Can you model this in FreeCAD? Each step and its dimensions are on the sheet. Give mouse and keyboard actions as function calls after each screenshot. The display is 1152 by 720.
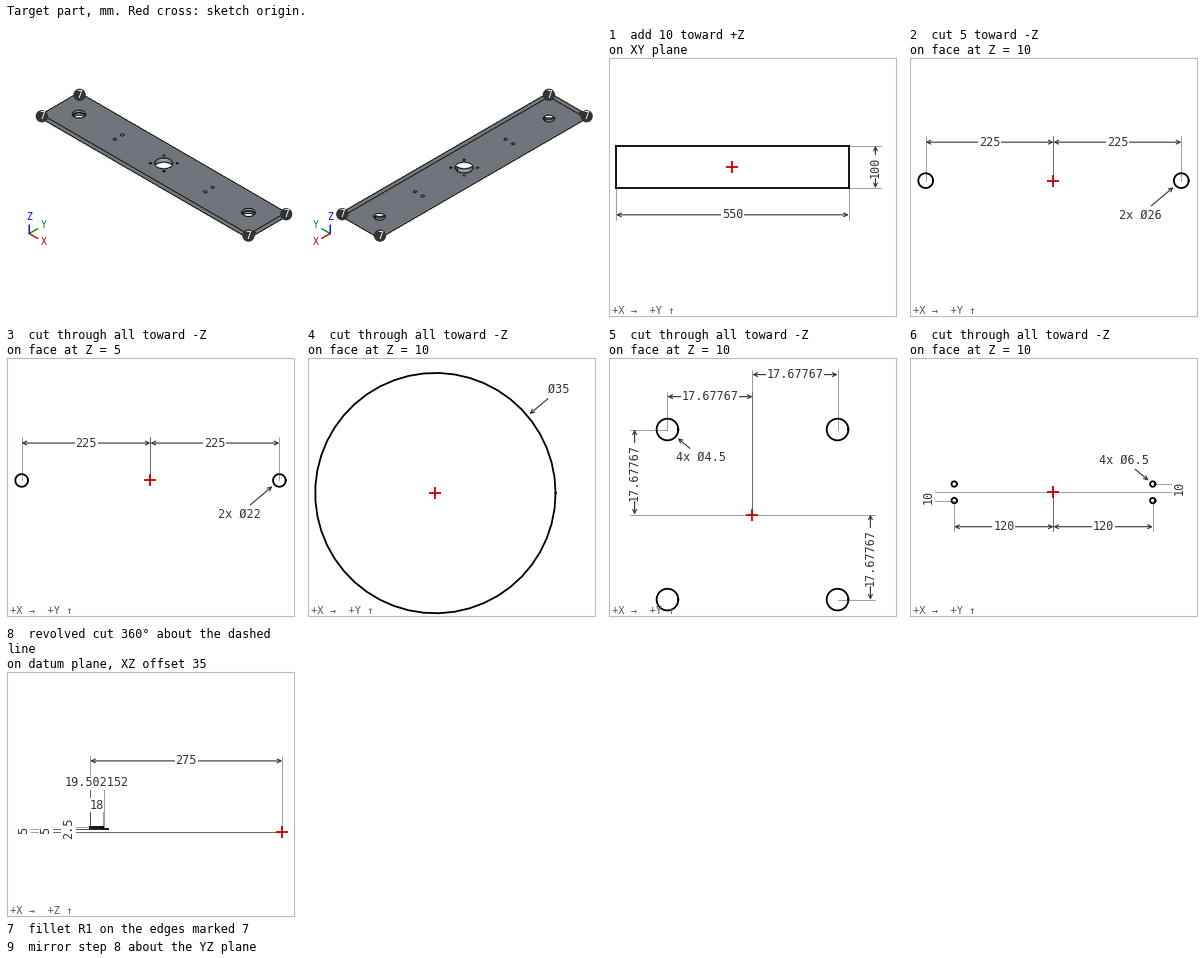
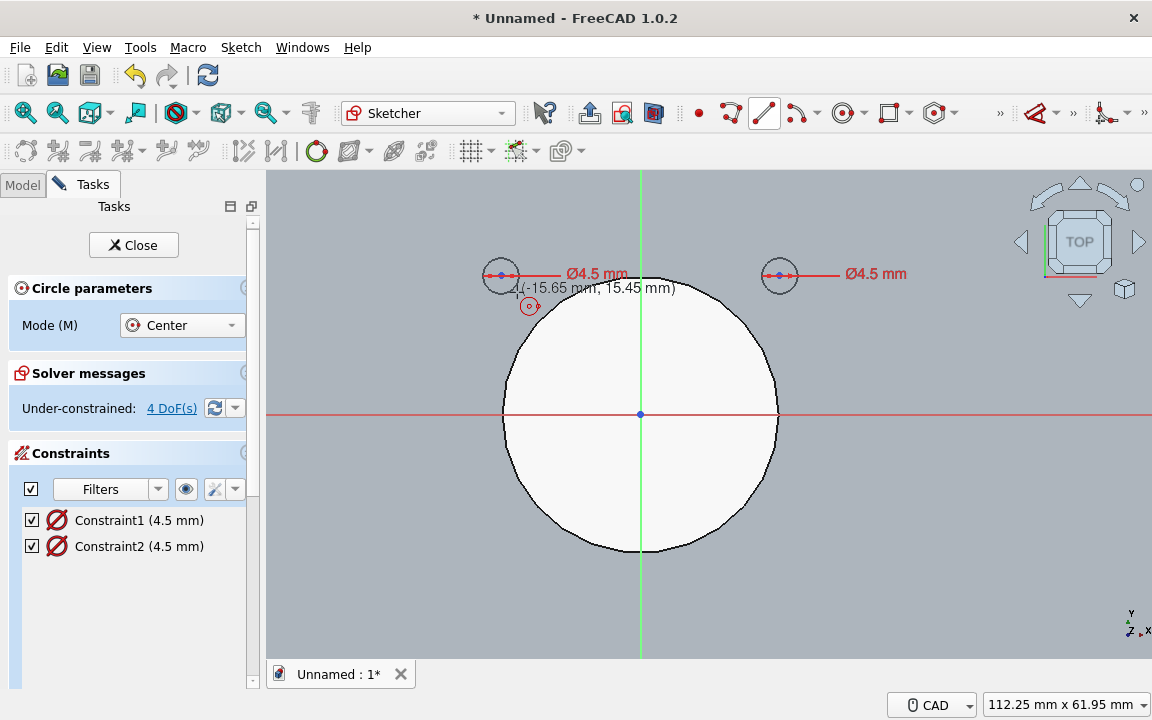
scroll(780, 554, up, 2)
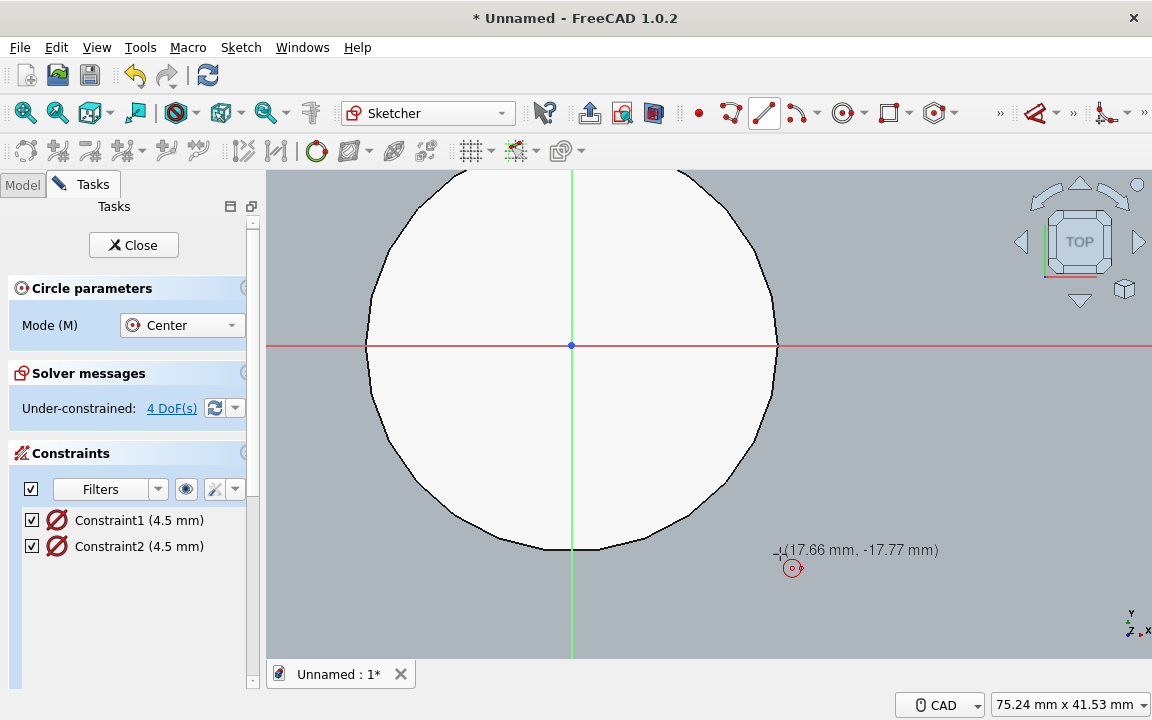
click(780, 554)
move(799, 535)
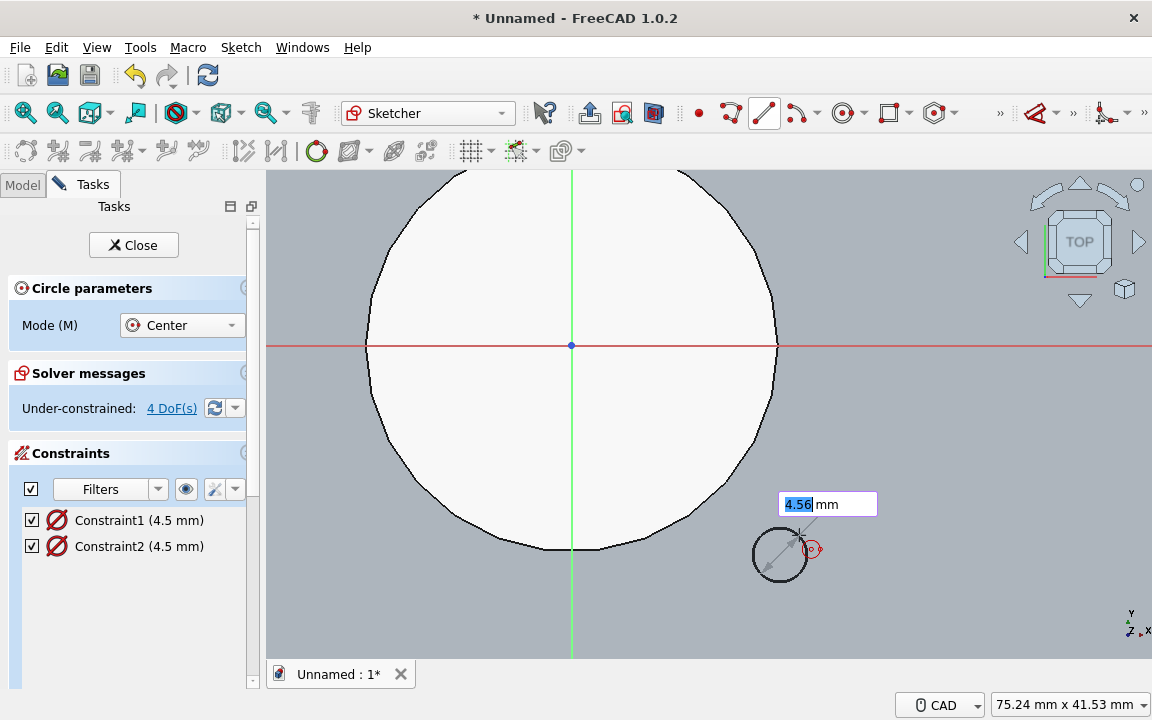
text(4.5)
key(Return)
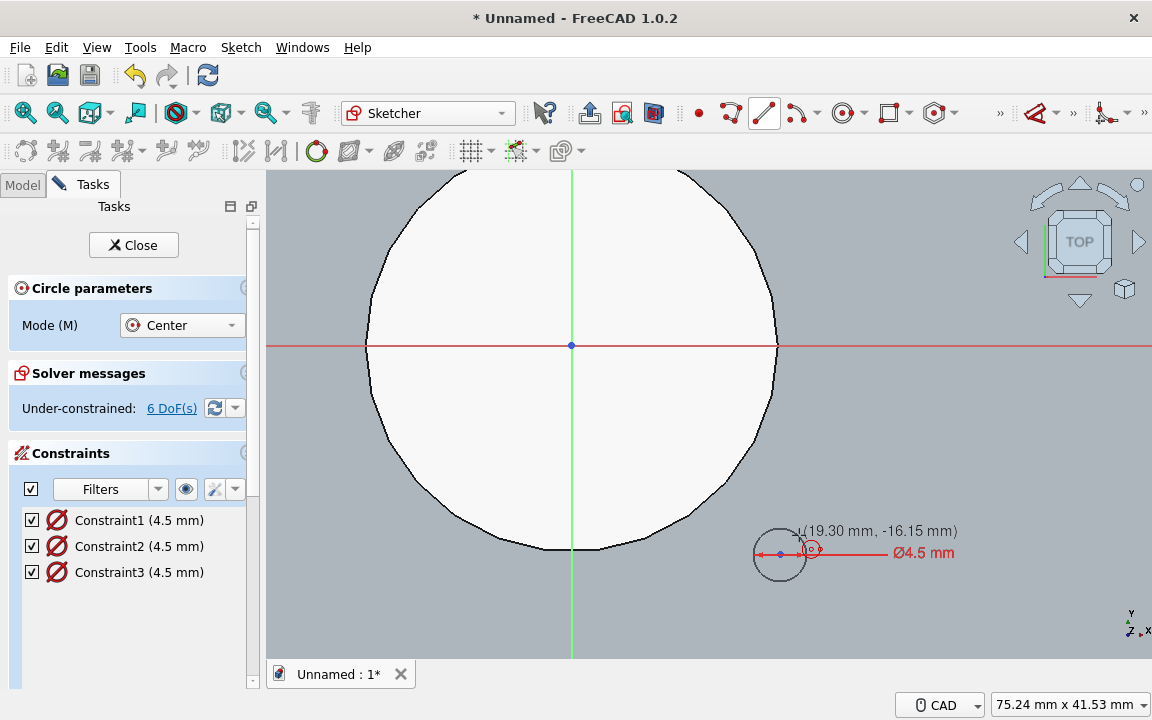
click(364, 554)
move(382, 535)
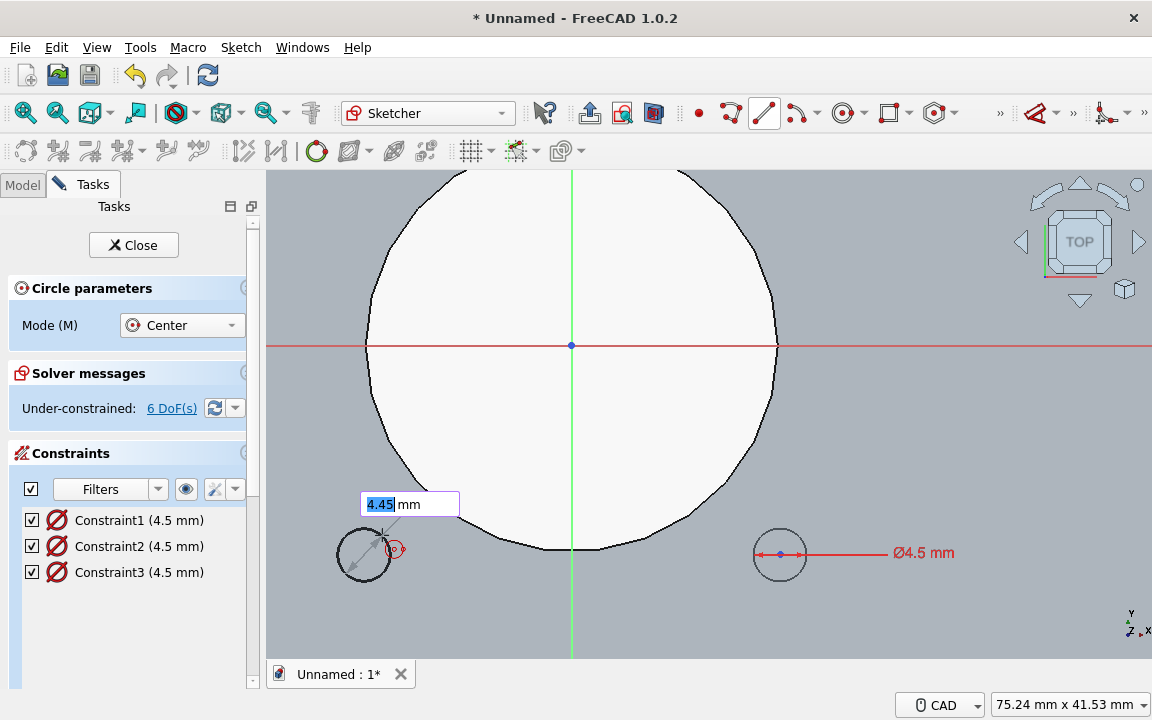
text(4.5)
key(Return)
key(Escape)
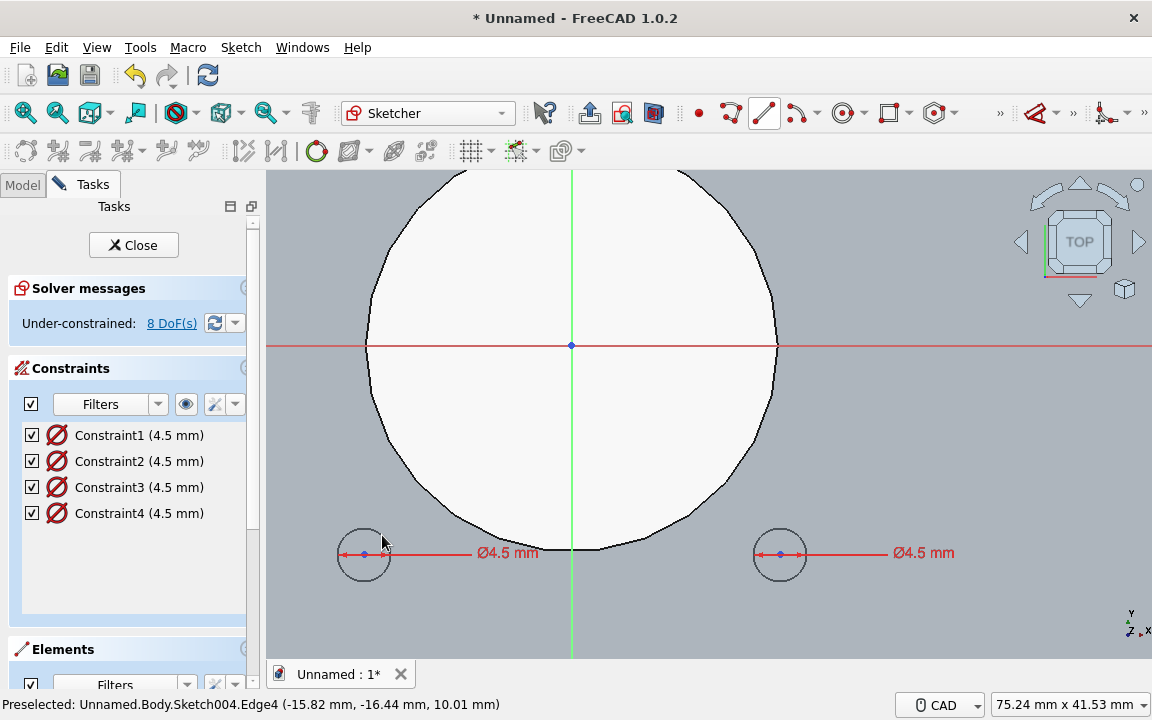
scroll(780, 554, down, 2)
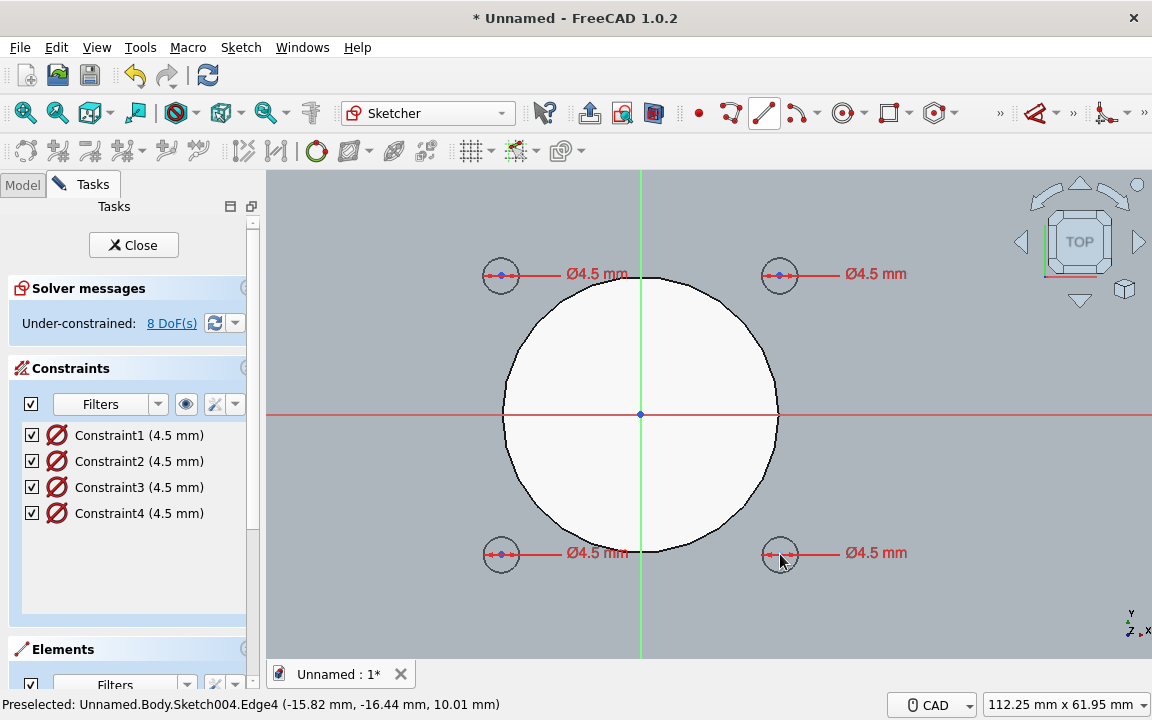
click(501, 276)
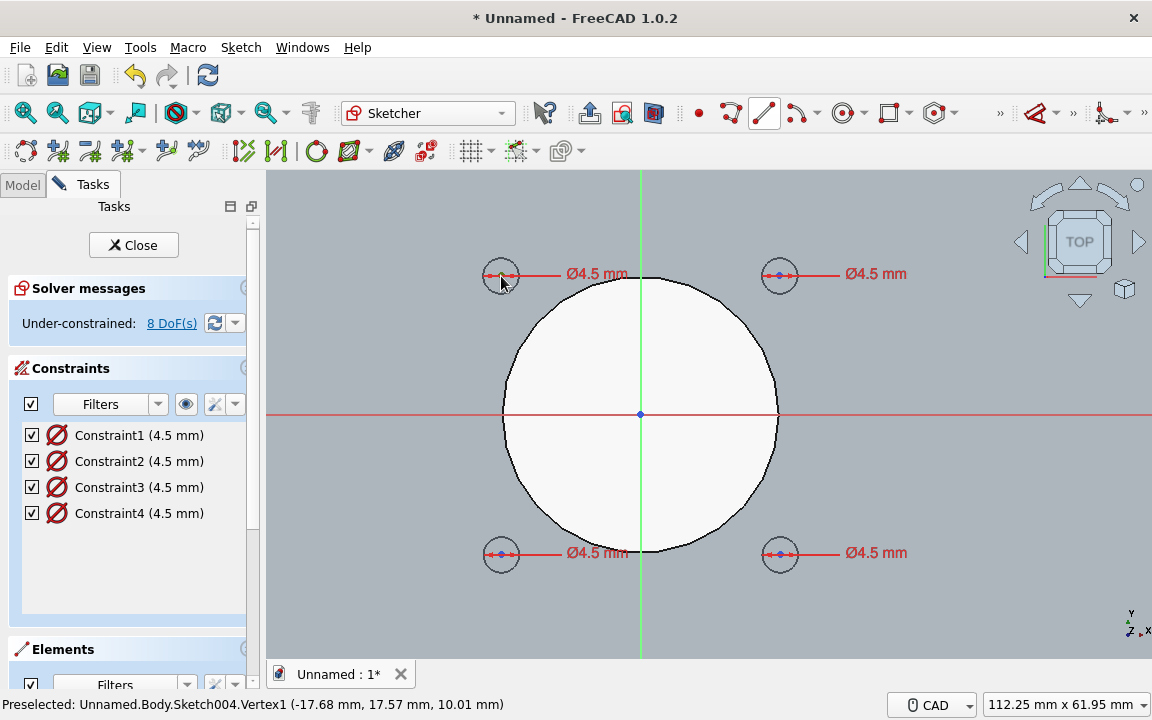
click(780, 276)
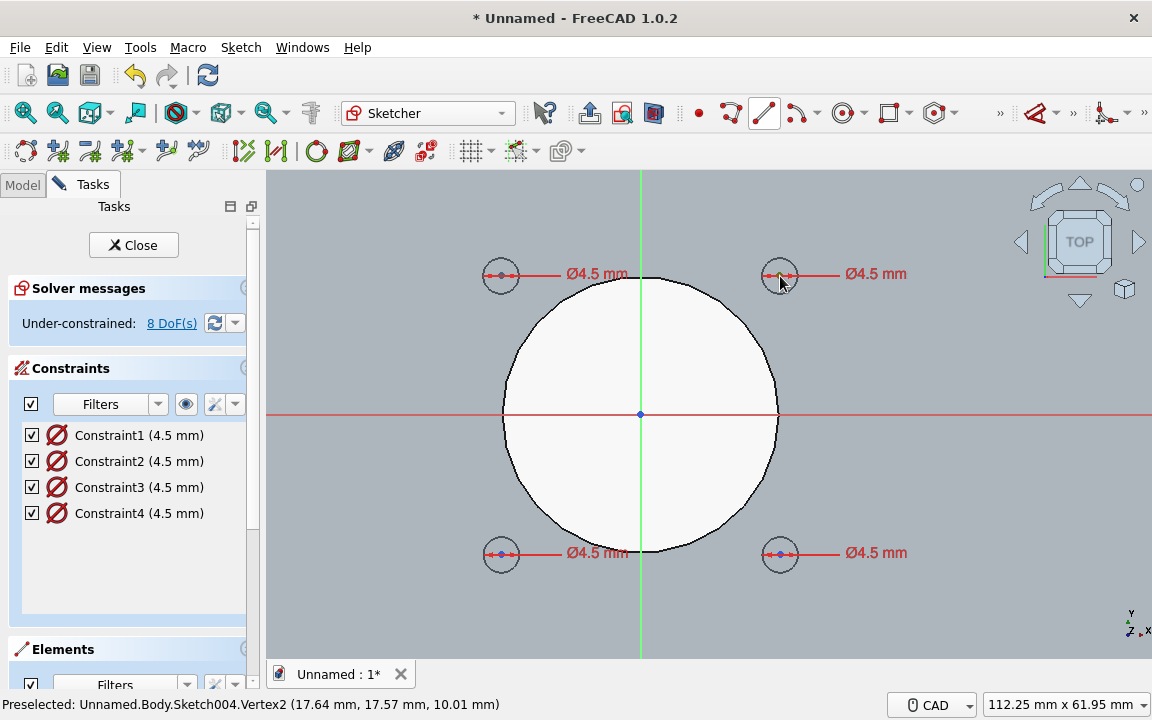
key(h)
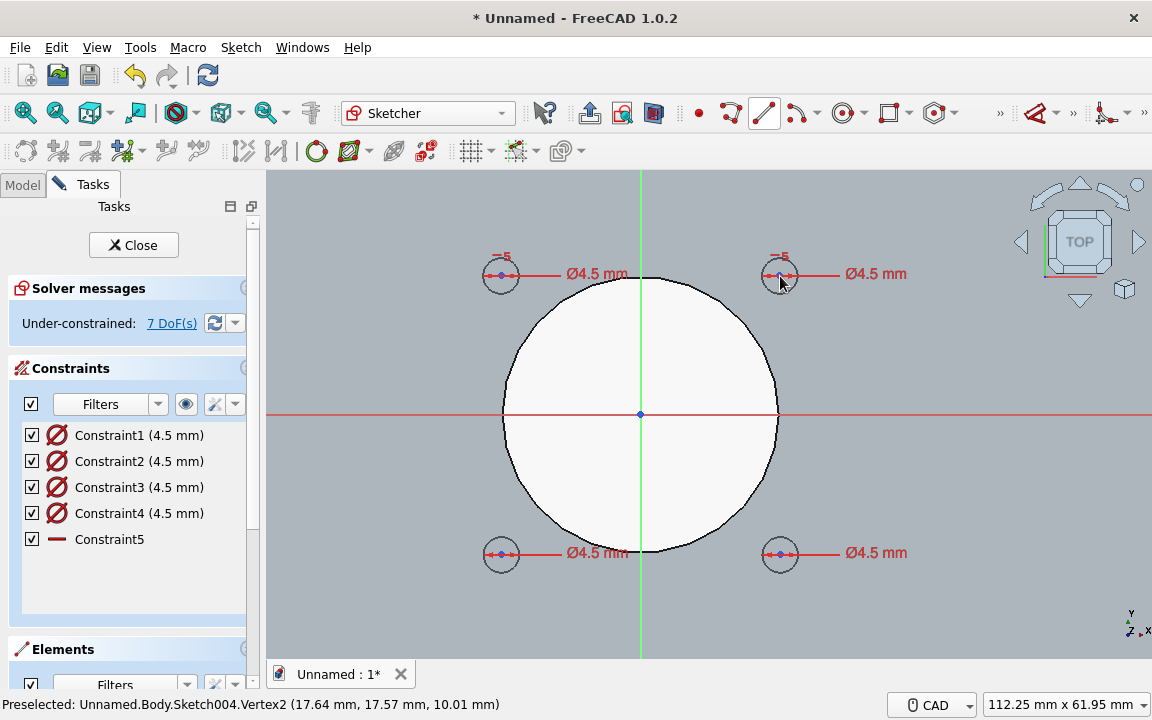
click(780, 276)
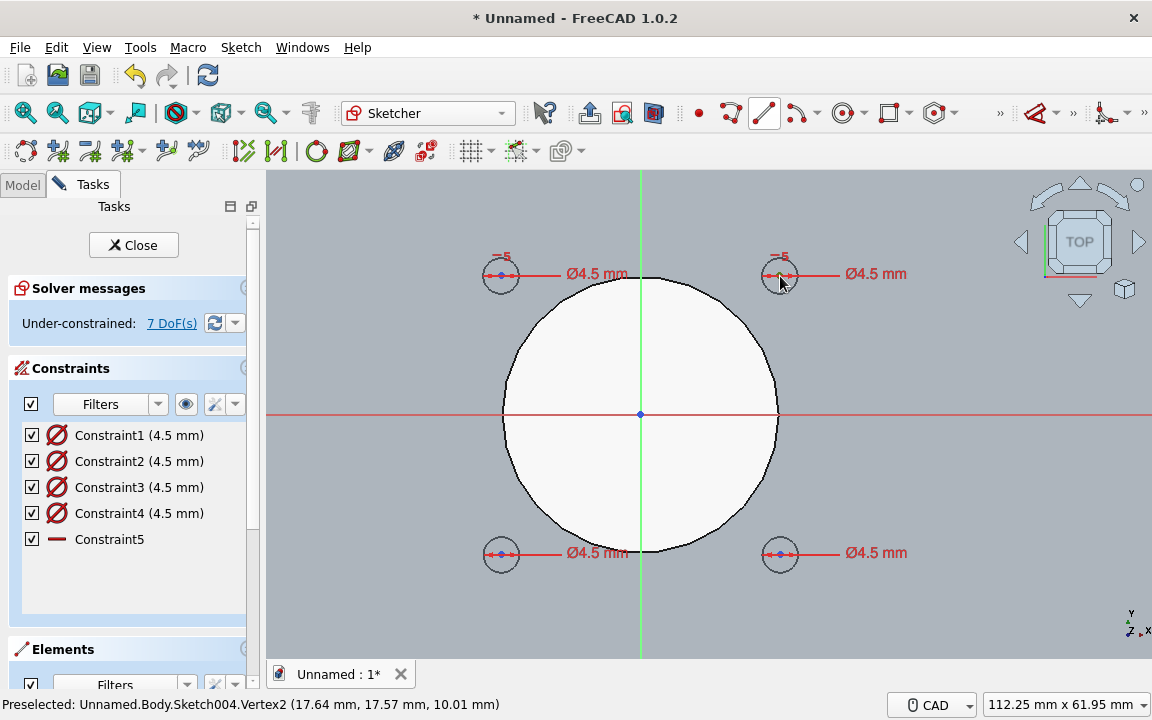
click(780, 555)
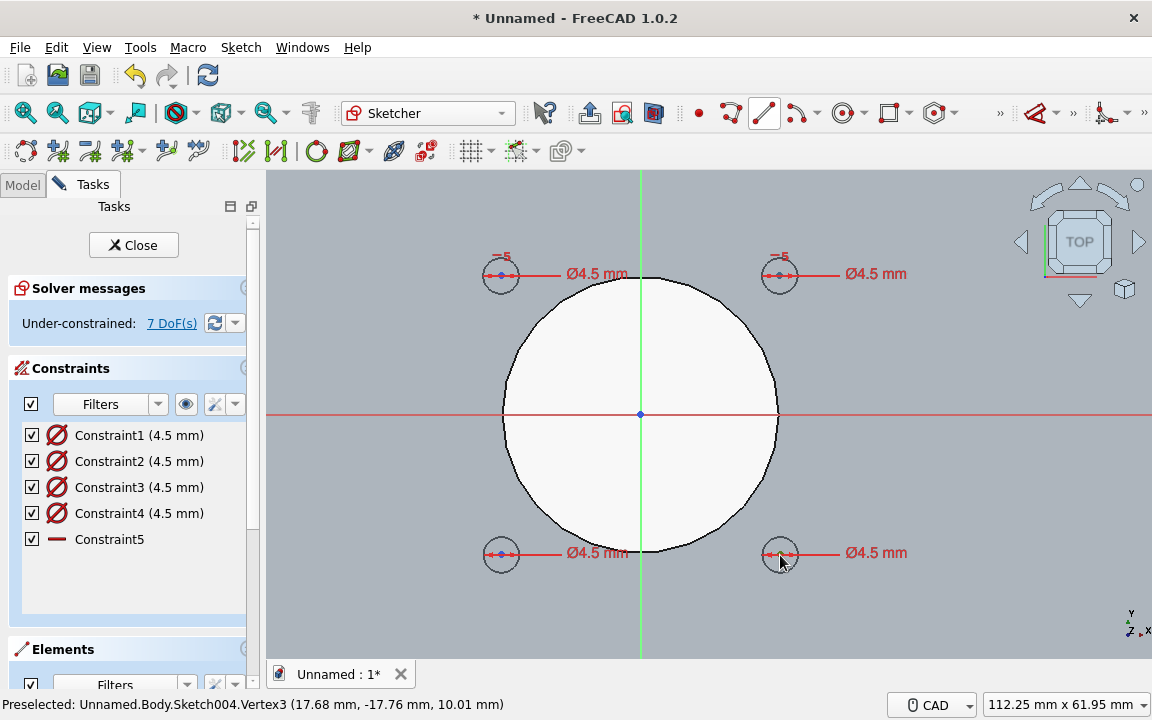
key(v)